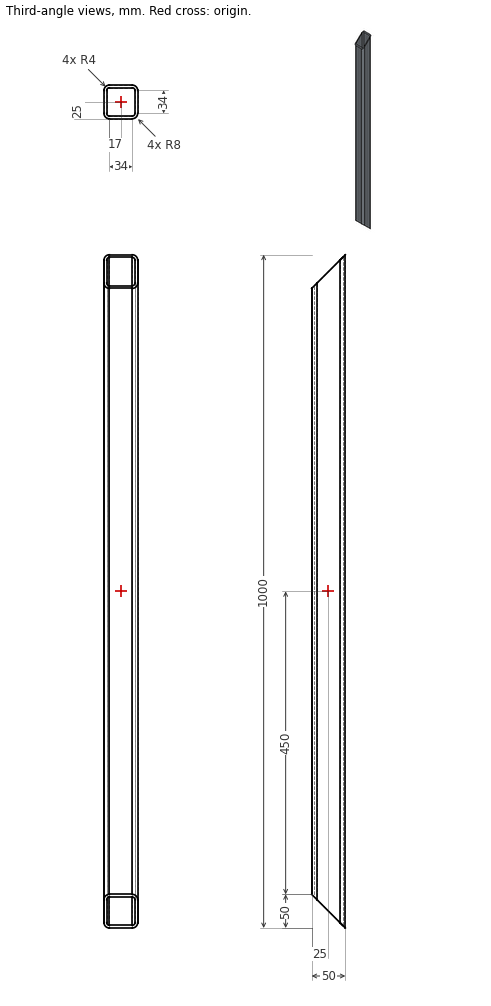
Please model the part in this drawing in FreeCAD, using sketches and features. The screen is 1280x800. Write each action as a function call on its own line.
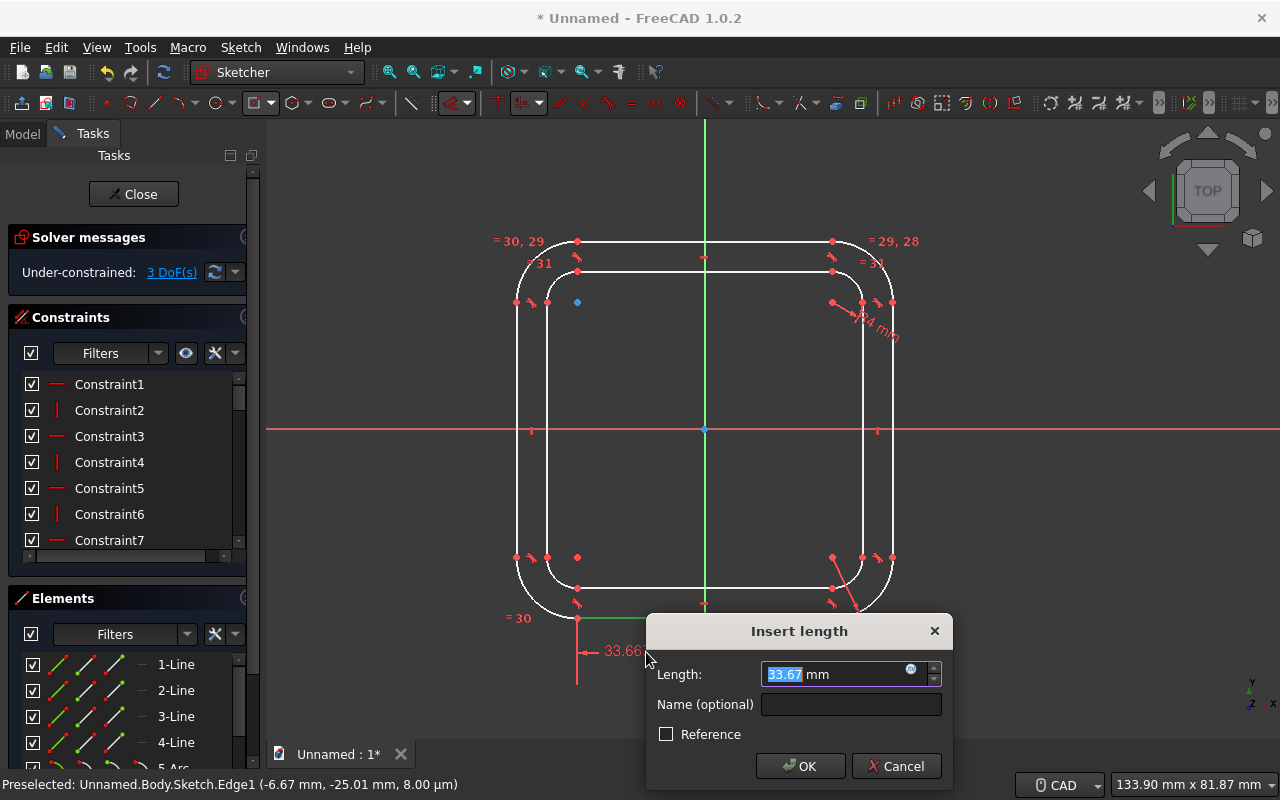
text(34)
key(Return)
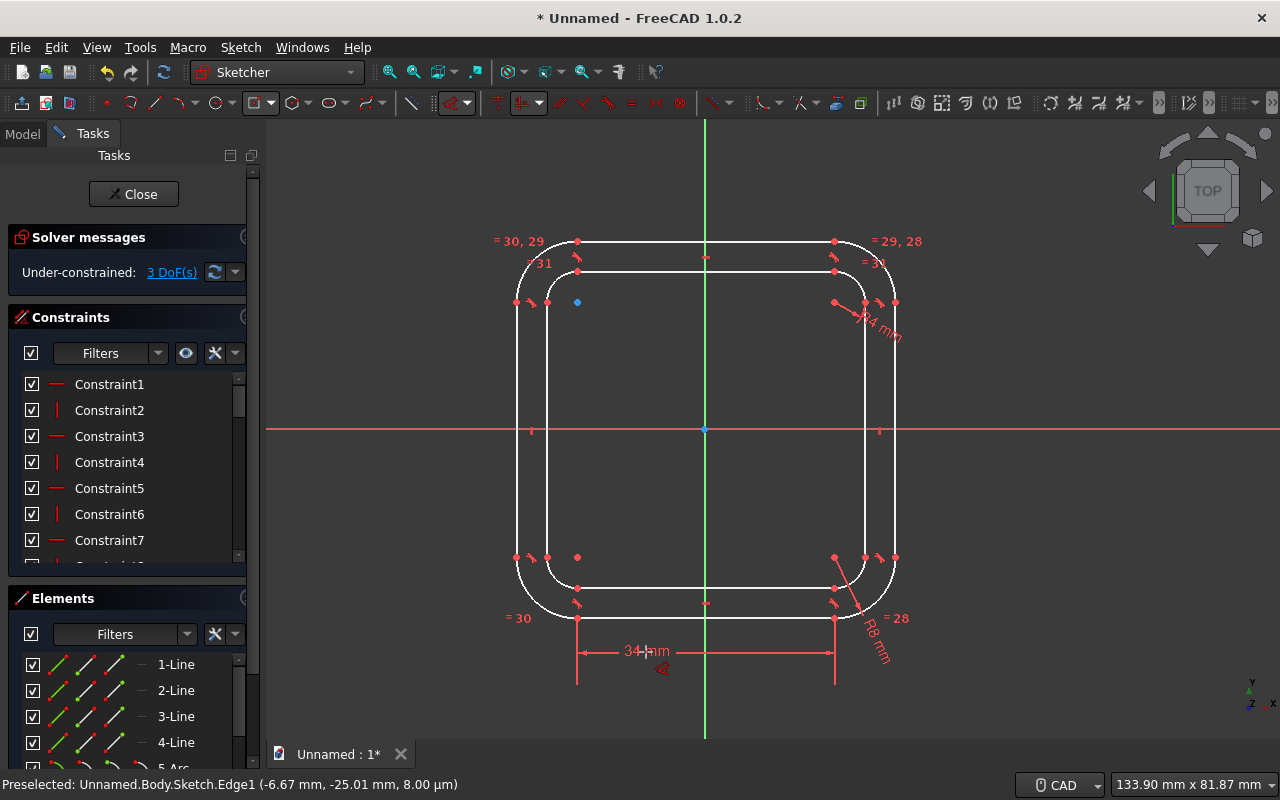
click(895, 481)
click(929, 371)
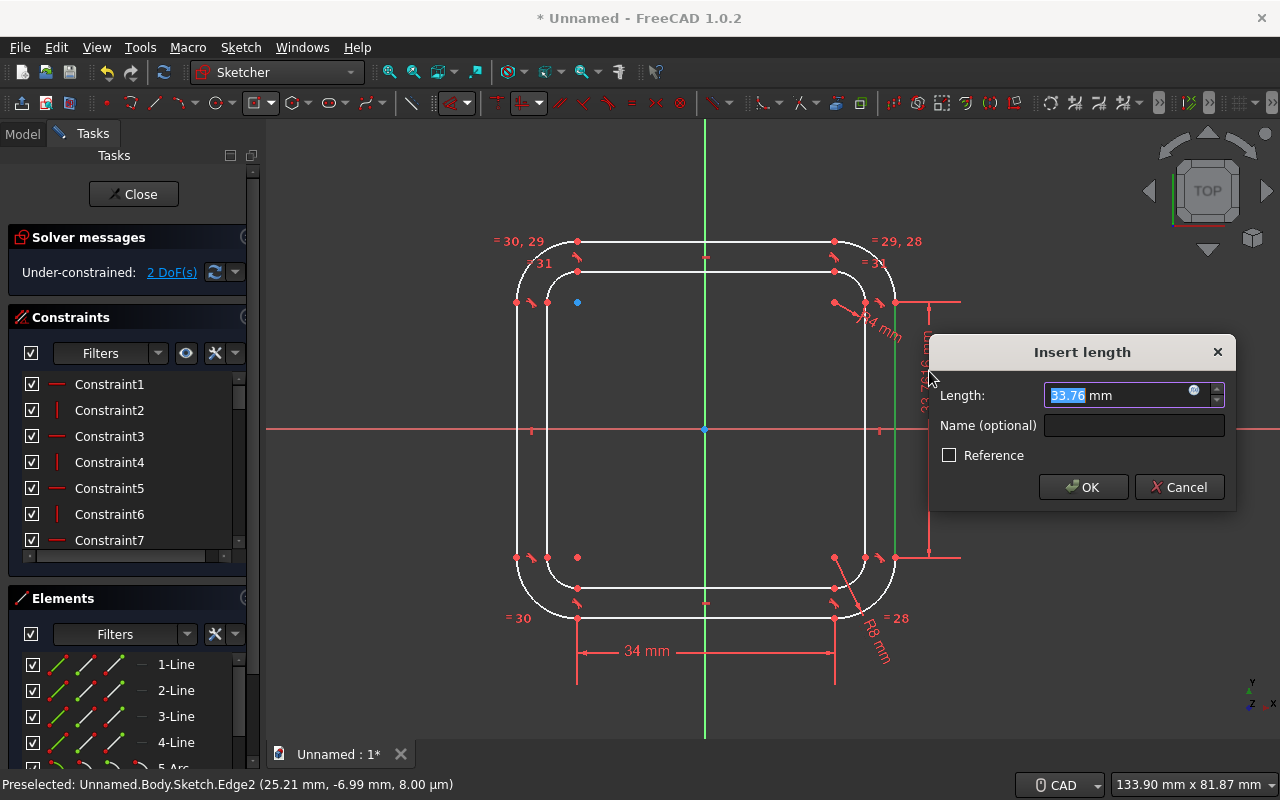
text(34)
key(Return)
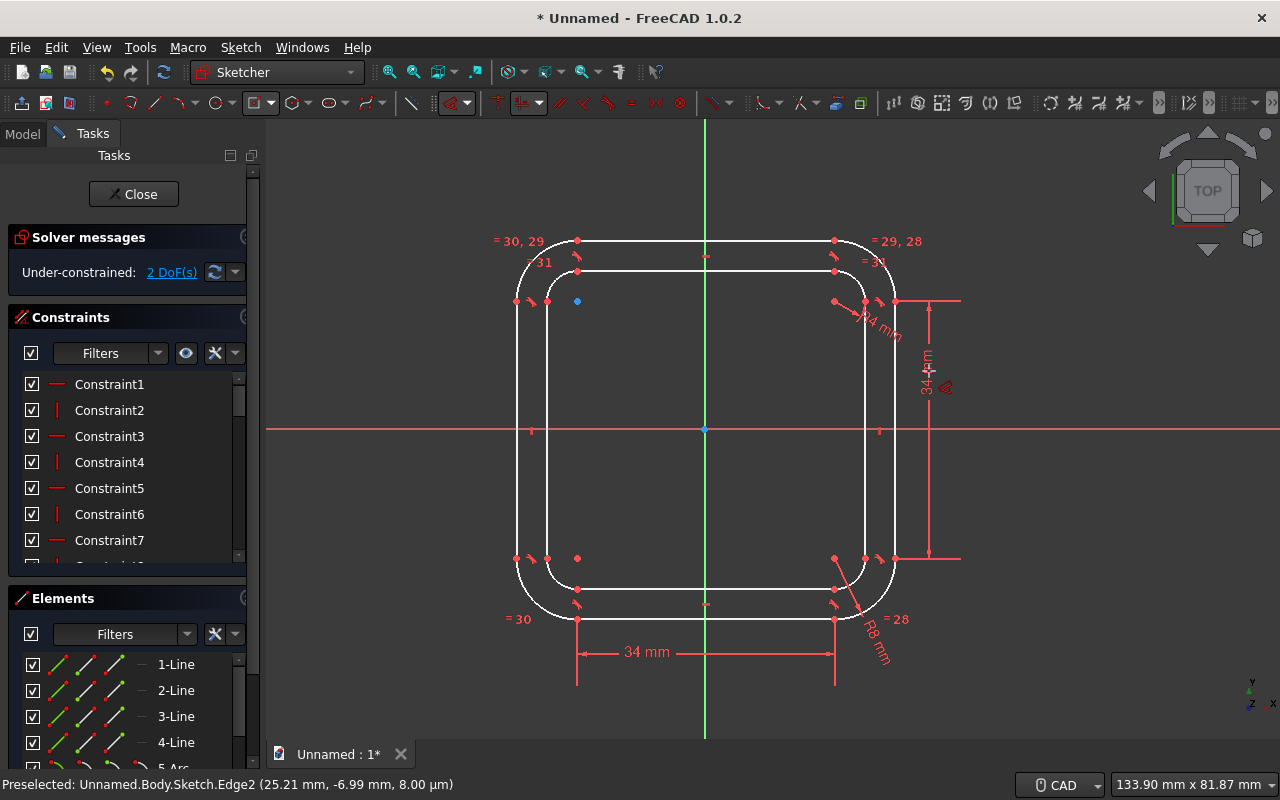
click(577, 619)
click(641, 395)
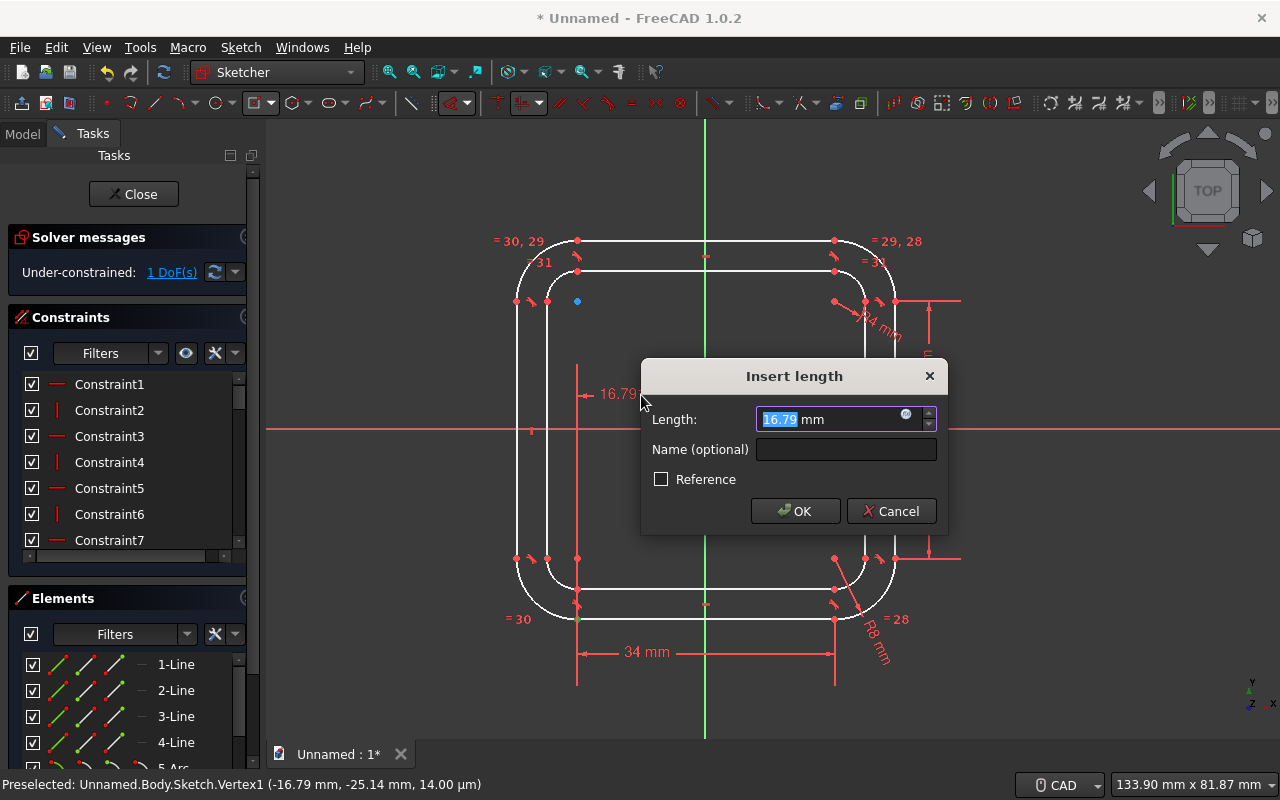
text(17)
key(Return)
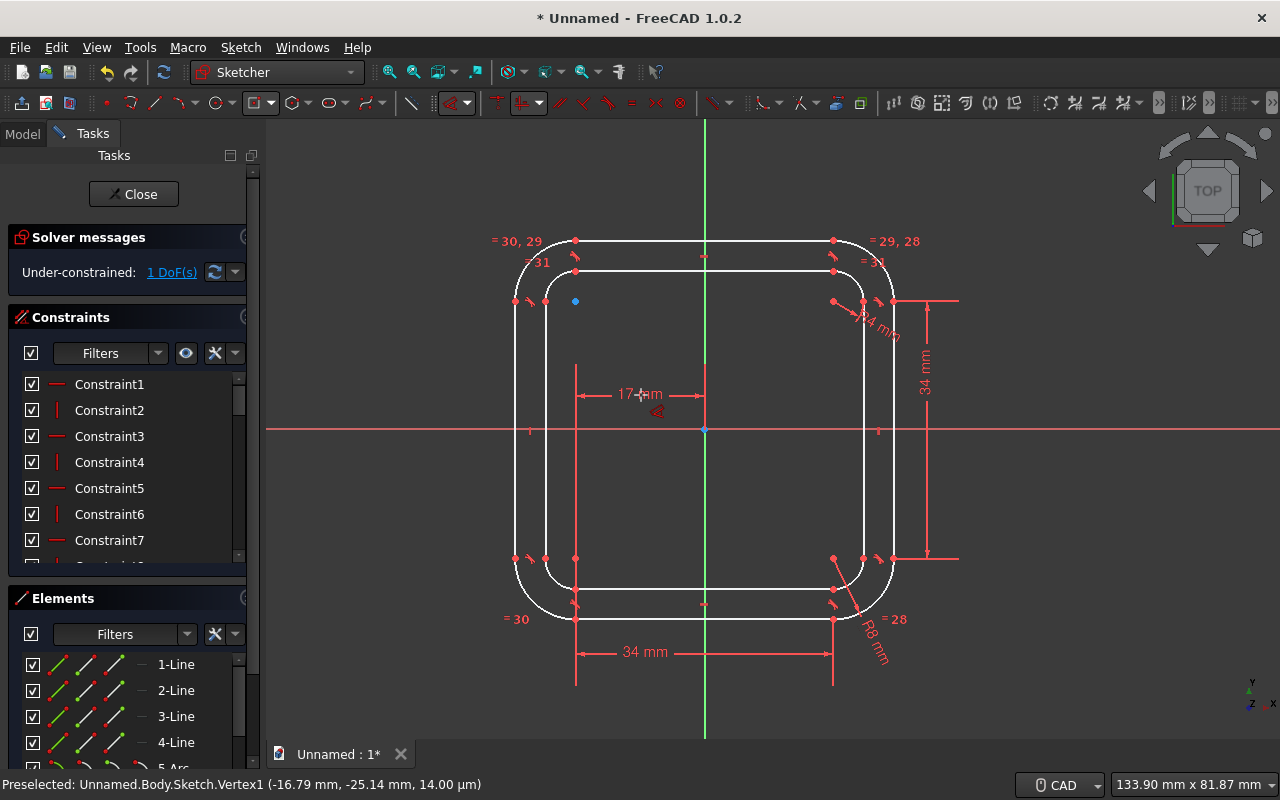
click(576, 619)
click(542, 591)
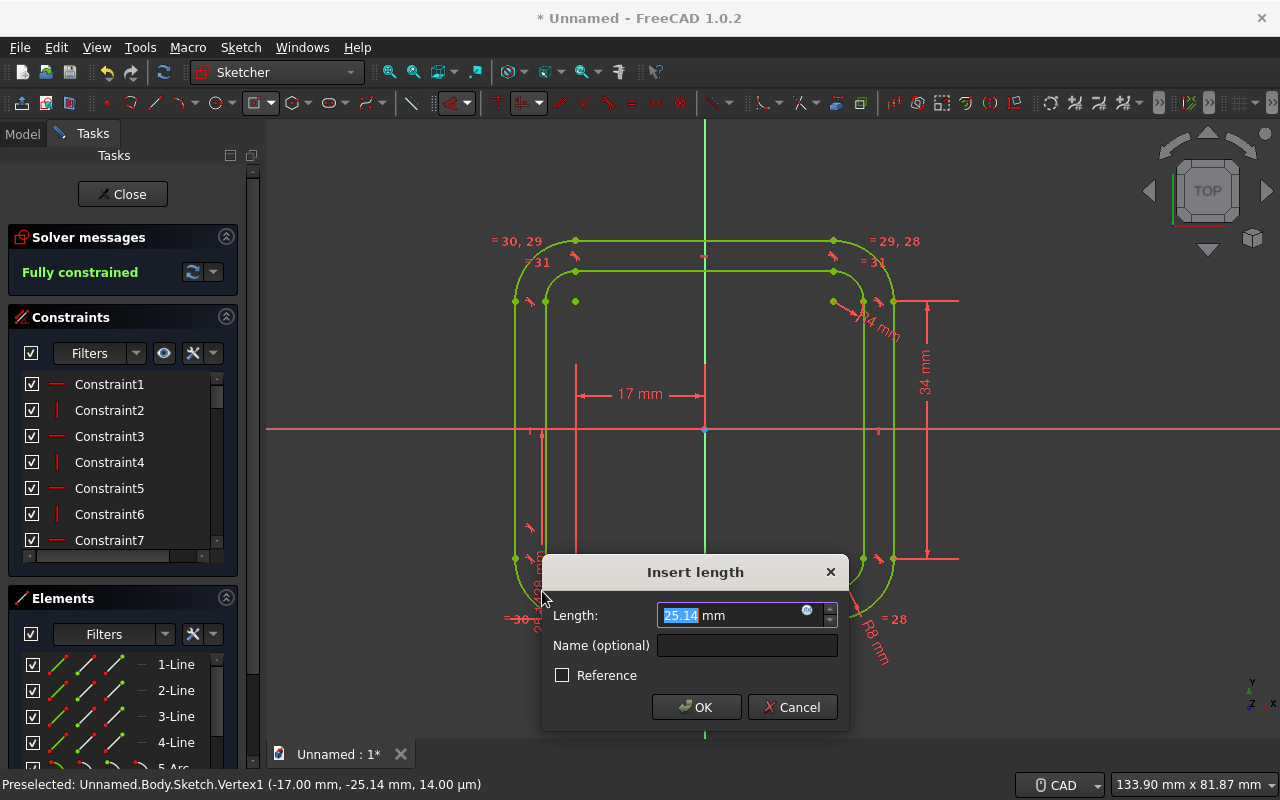
text(25)
key(Return)
key(Escape)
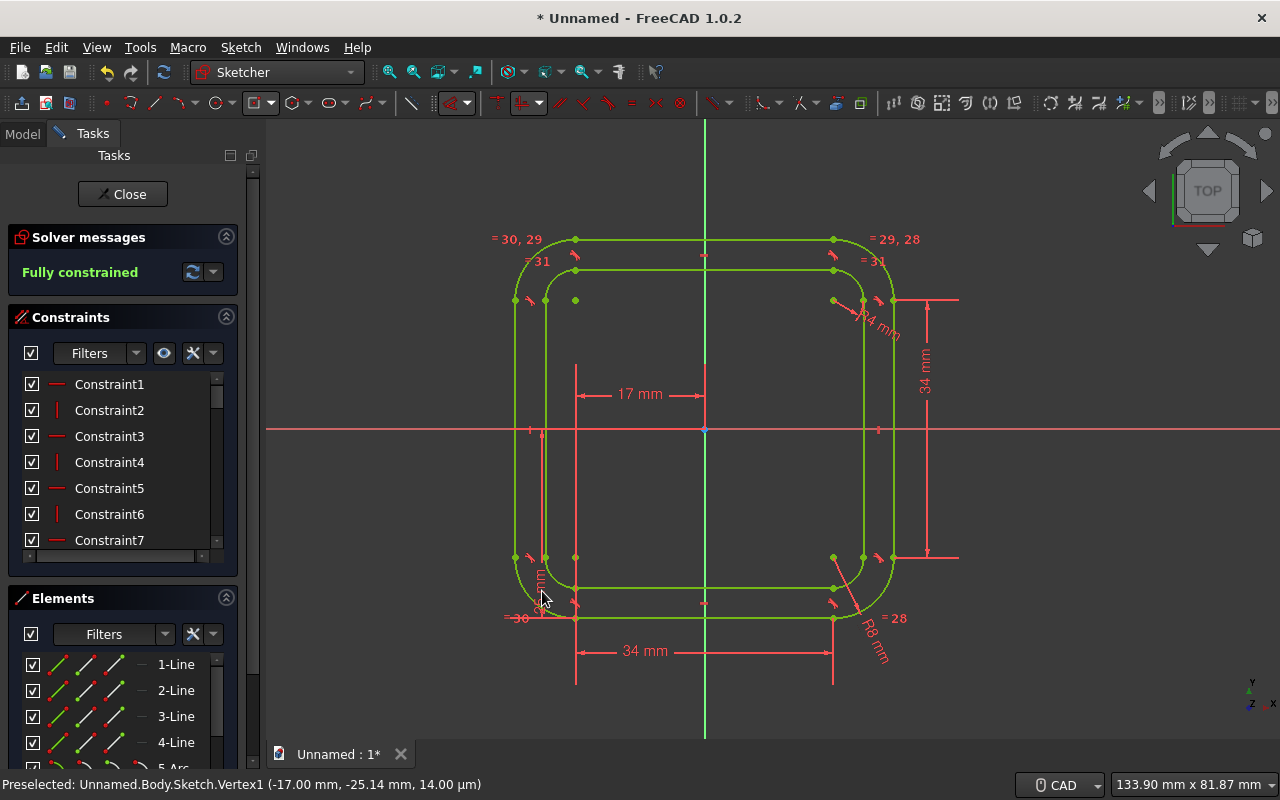
click(123, 194)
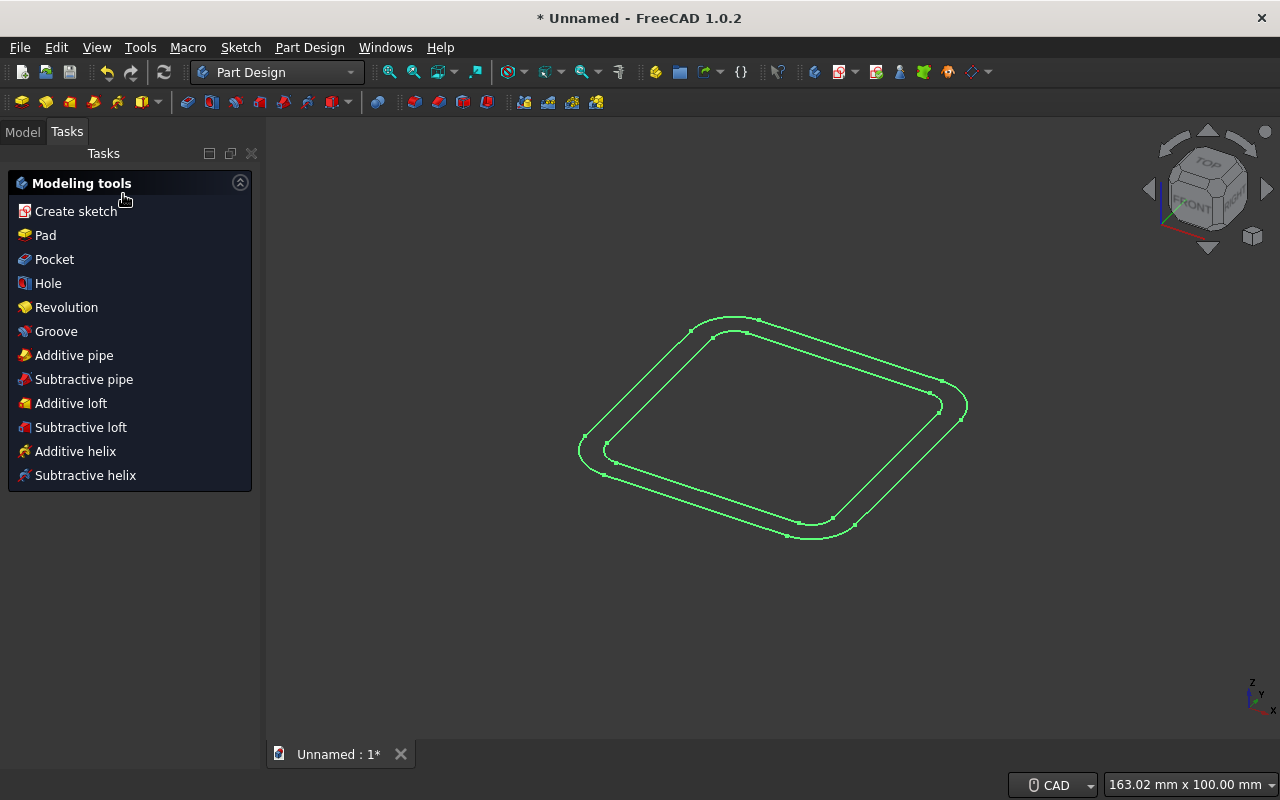
click(22, 102)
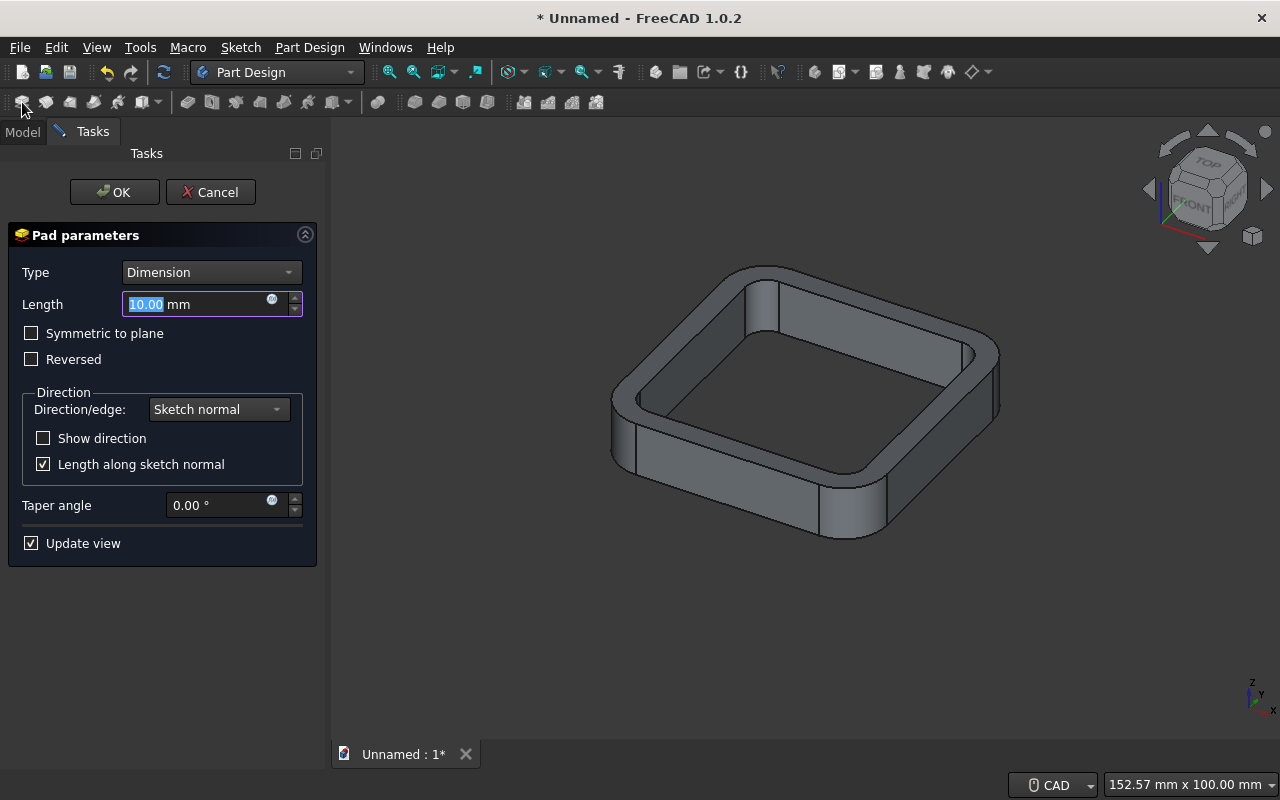
text(1000)
key(Tab)